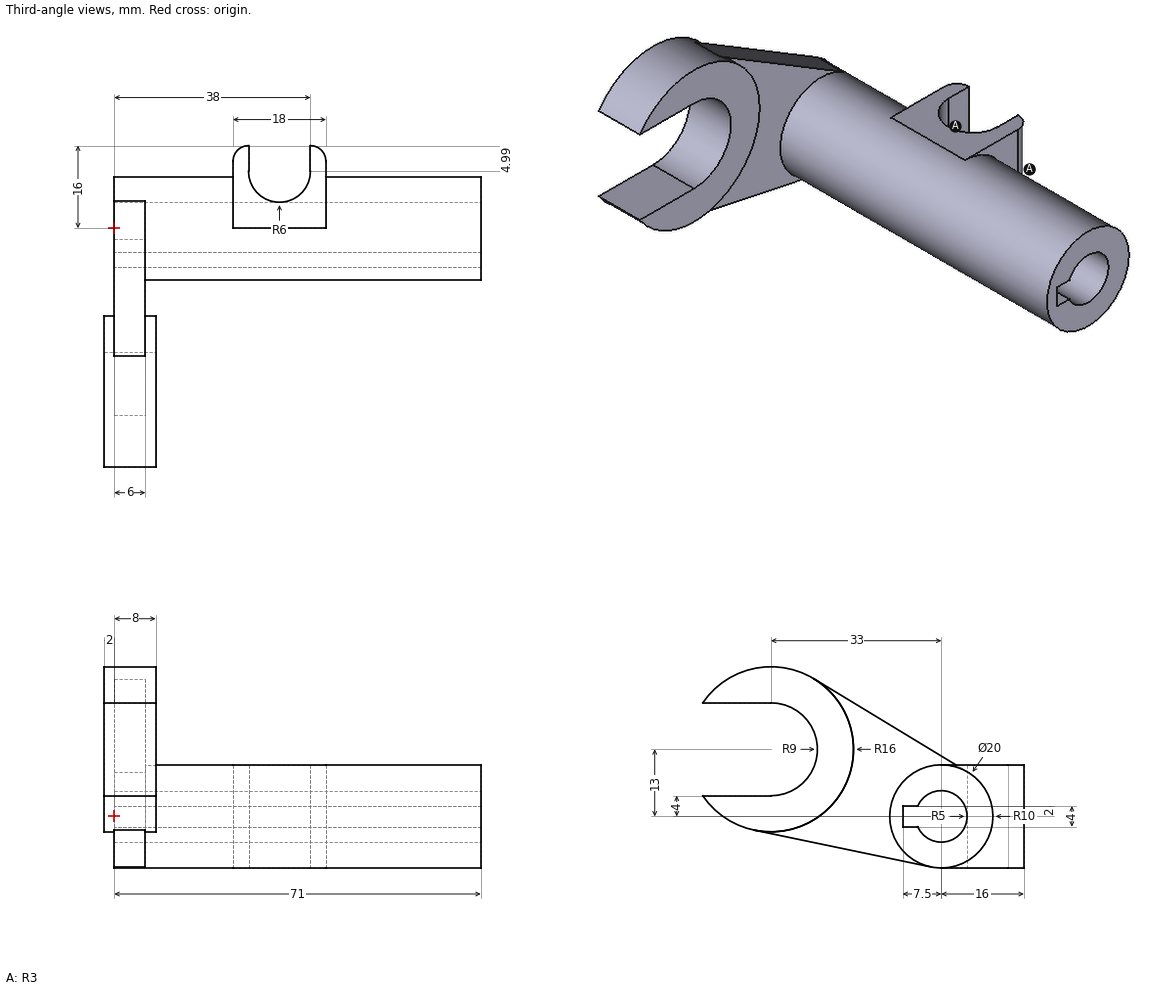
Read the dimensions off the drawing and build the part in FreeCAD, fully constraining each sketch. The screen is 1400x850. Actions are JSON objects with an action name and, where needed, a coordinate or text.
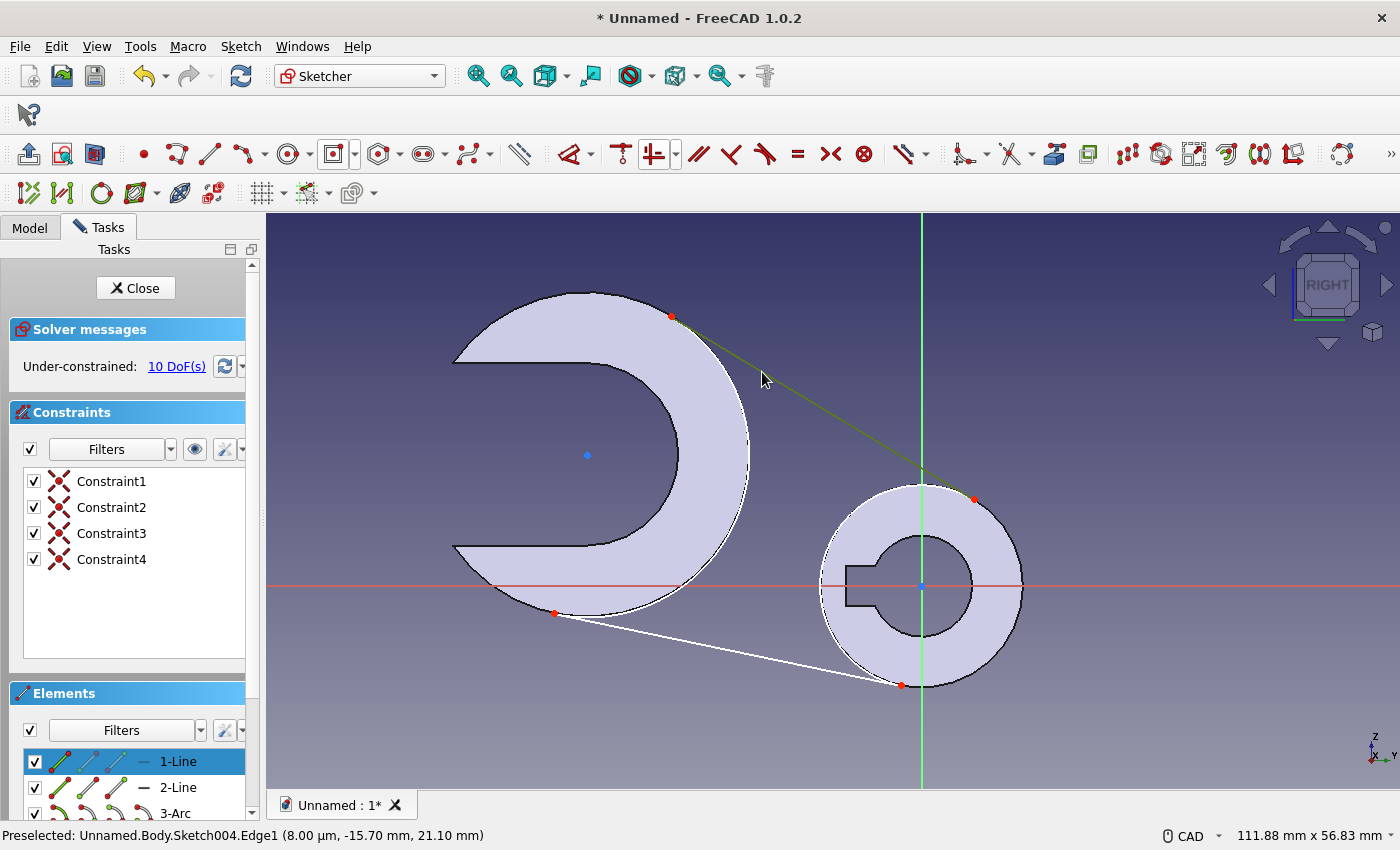
{"action": "left_click", "coordinate": [873, 498]}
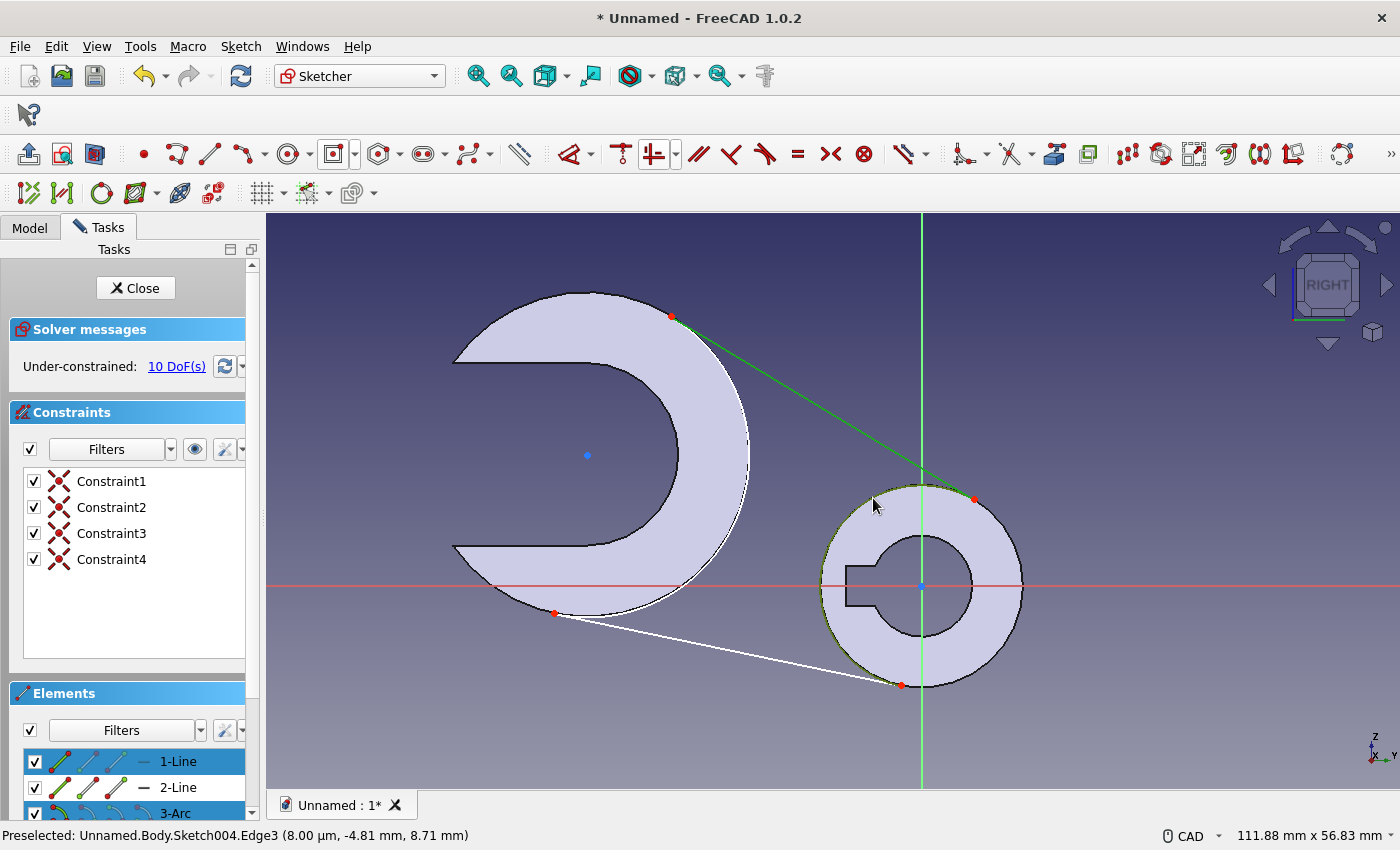
{"action": "key", "text": "t"}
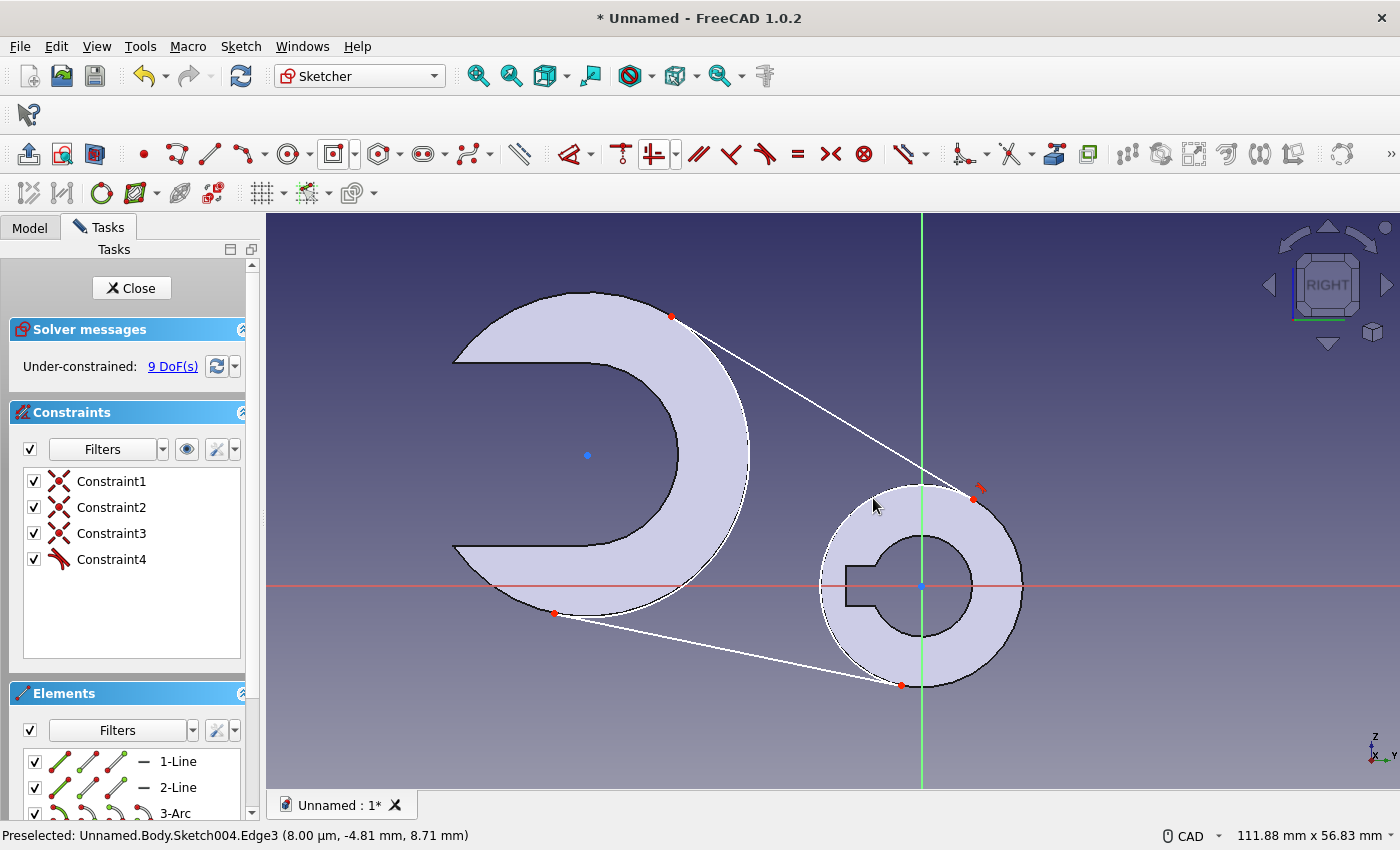
{"action": "left_click", "coordinate": [762, 372]}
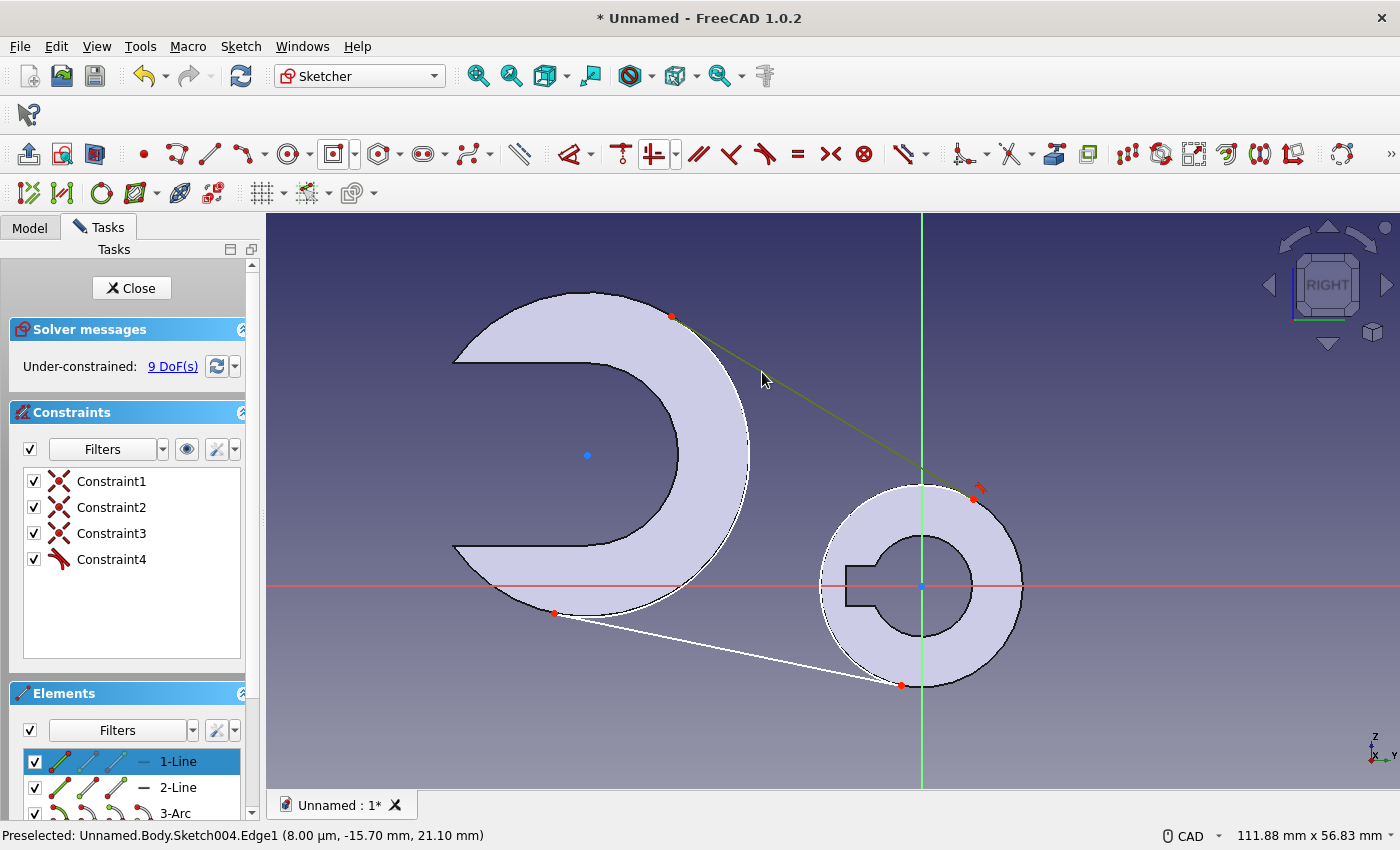
{"action": "left_click", "coordinate": [683, 586]}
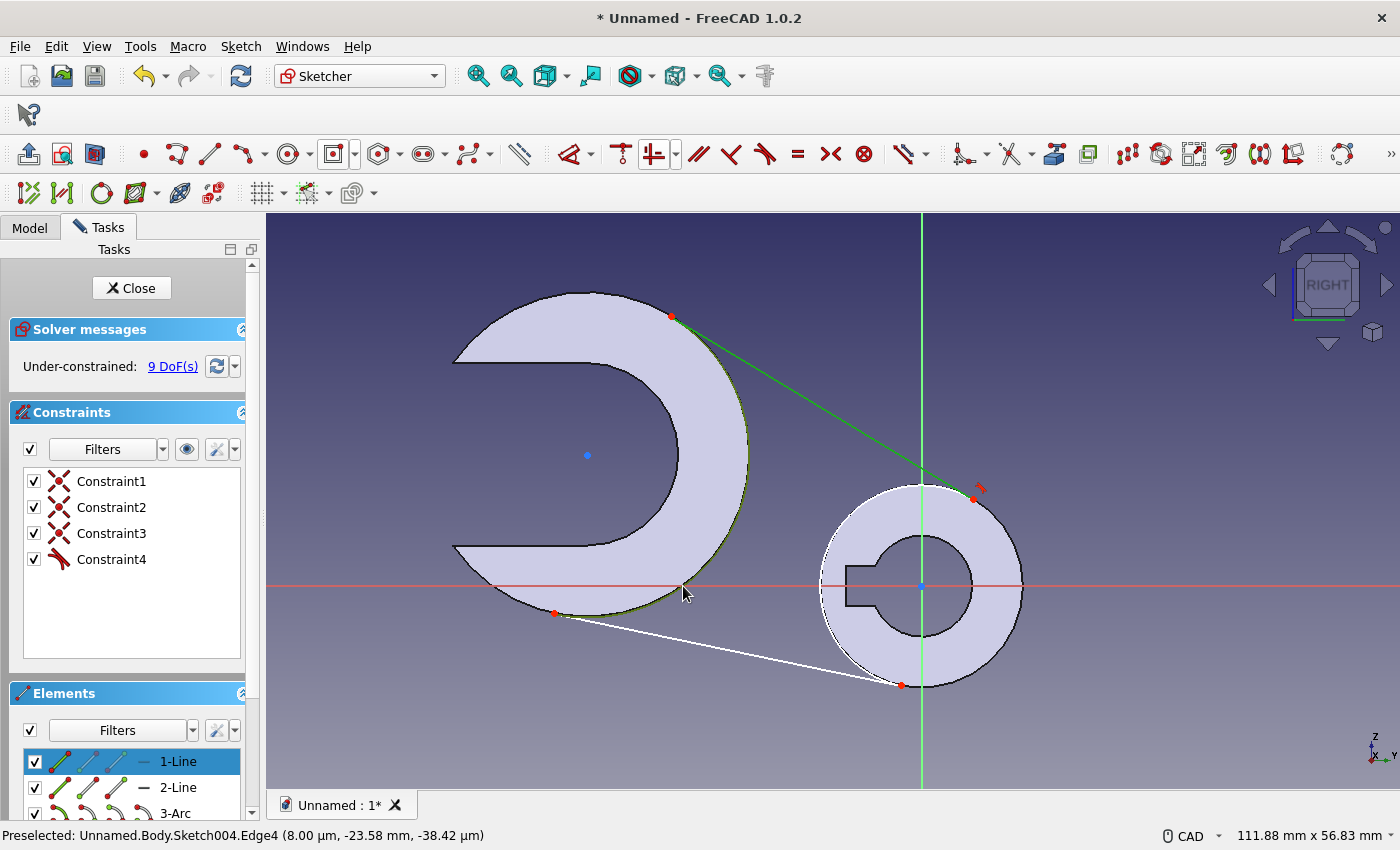
{"action": "key", "text": "t"}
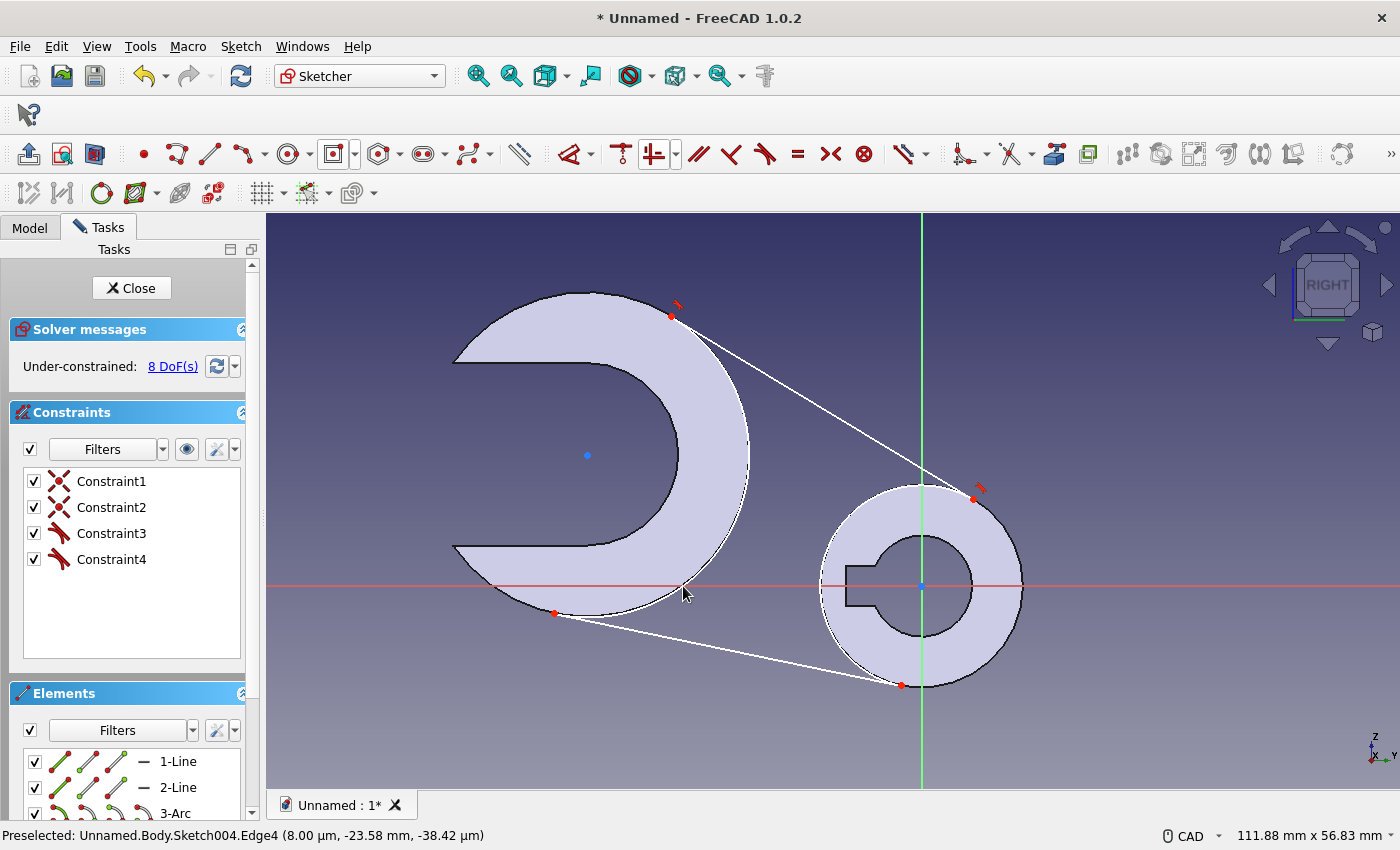
{"action": "left_click", "coordinate": [797, 664]}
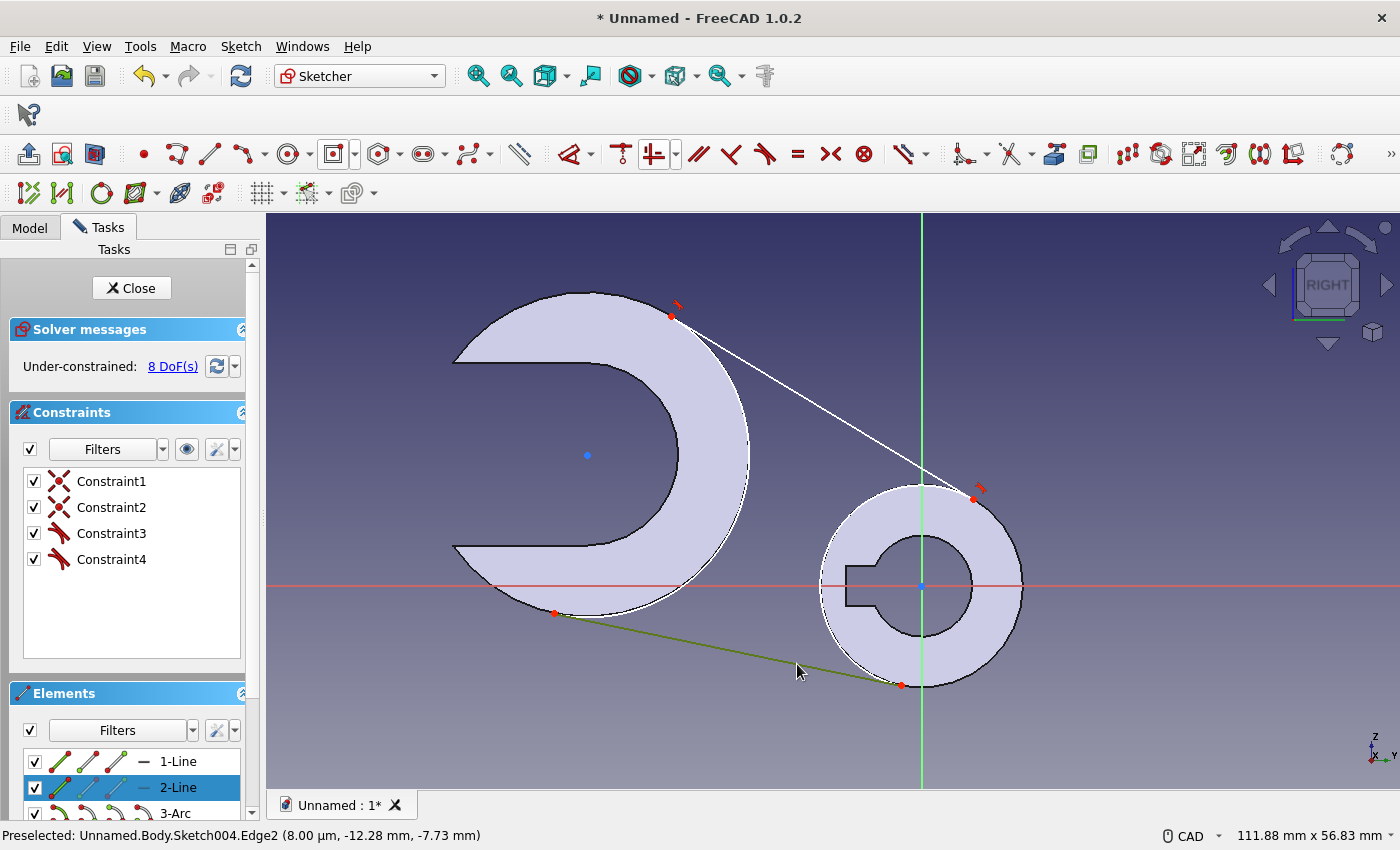
{"action": "left_click", "coordinate": [873, 498]}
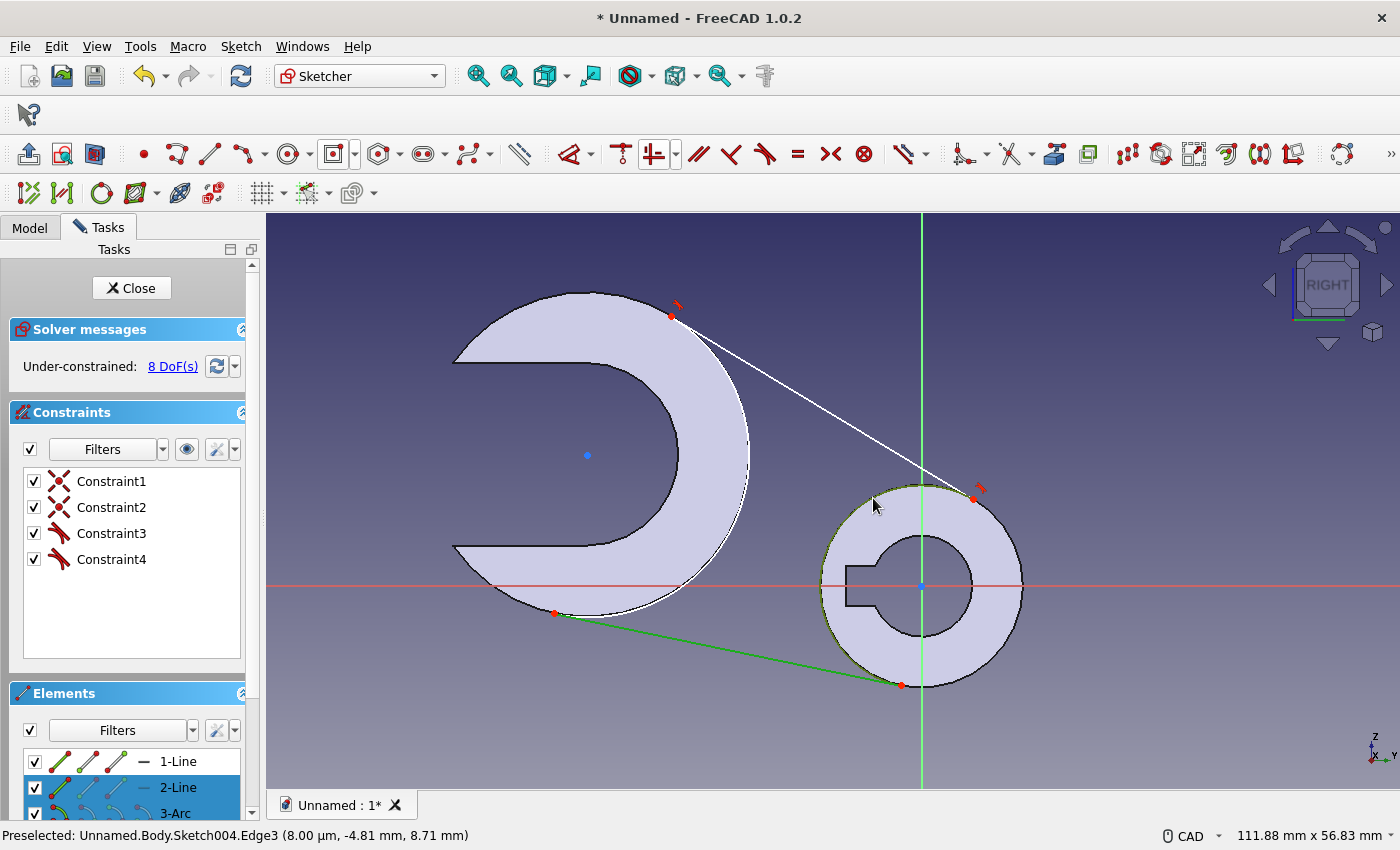
{"action": "key", "text": "t"}